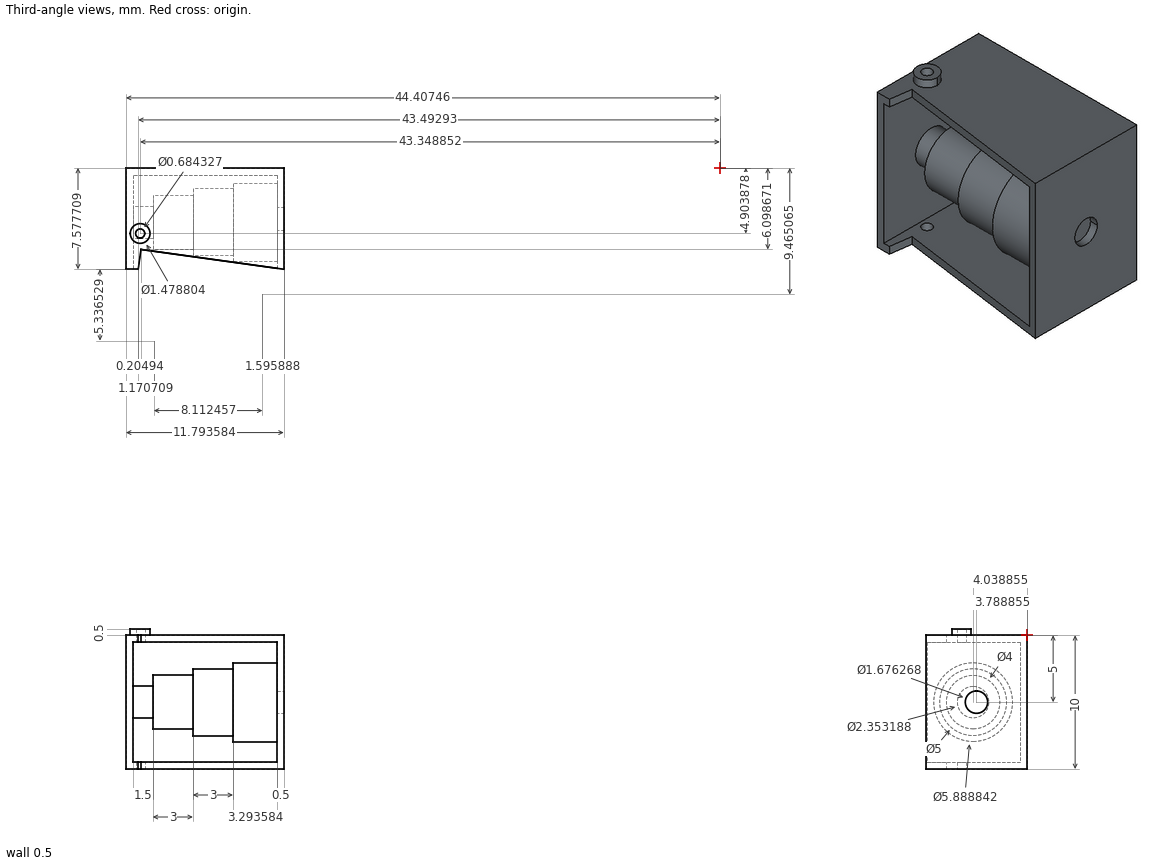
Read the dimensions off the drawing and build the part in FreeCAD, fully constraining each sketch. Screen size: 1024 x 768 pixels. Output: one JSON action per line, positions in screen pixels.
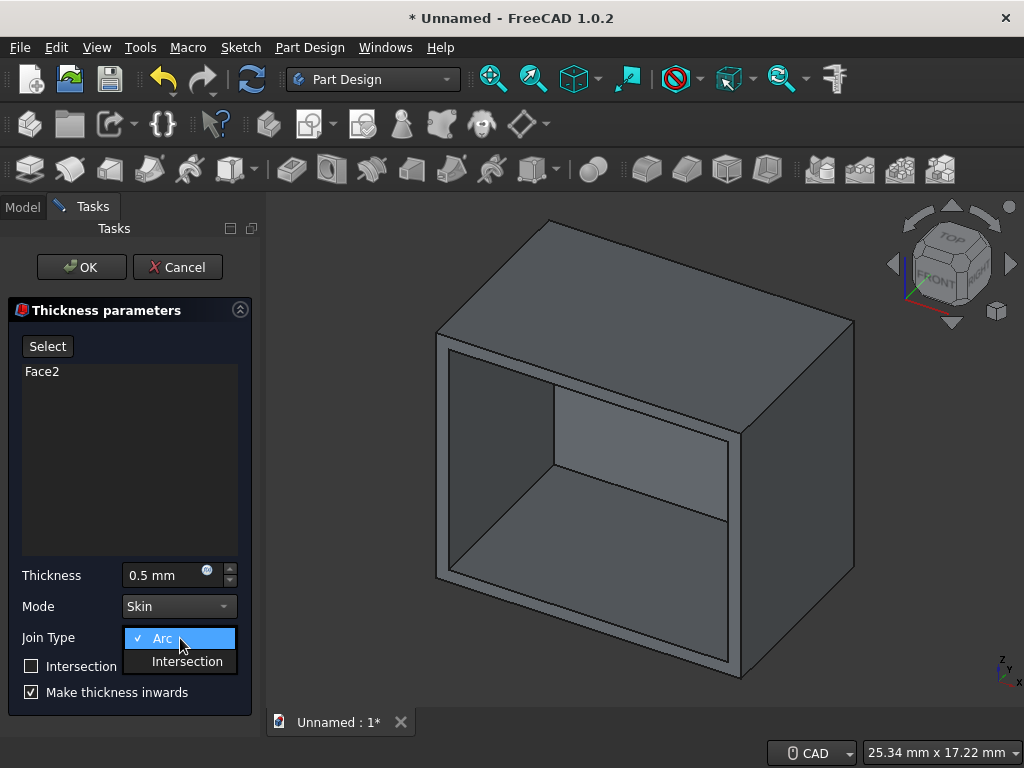
{"action": "left_click", "coordinate": [179, 662]}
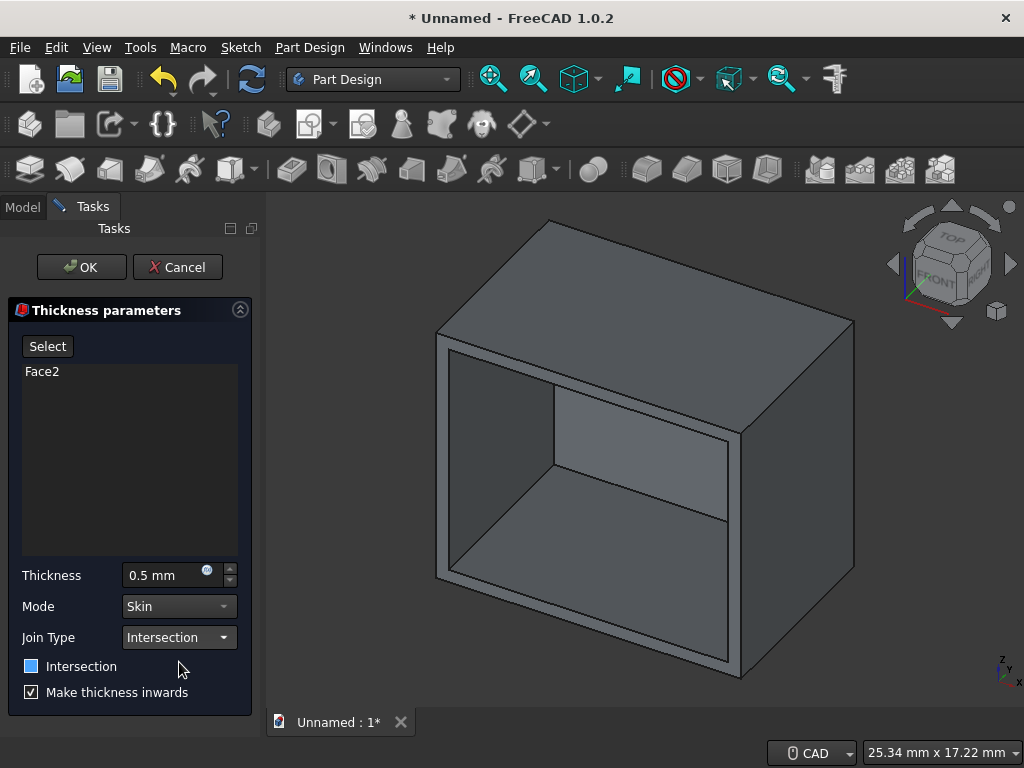
{"action": "left_click", "coordinate": [82, 267]}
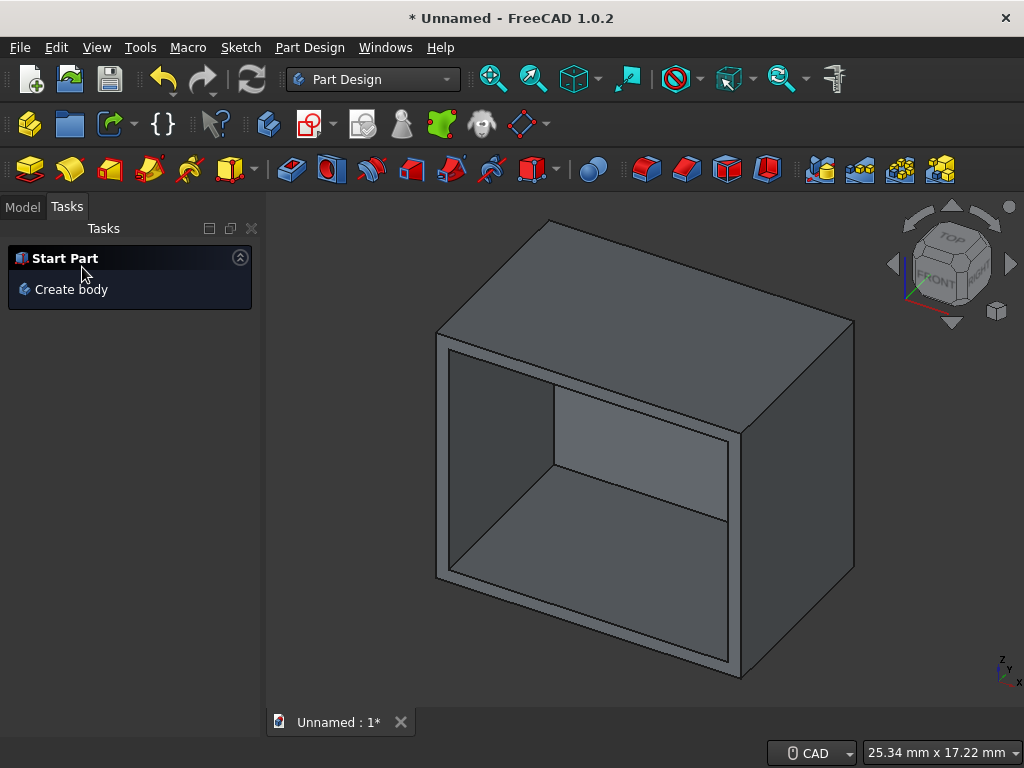
{"action": "left_click", "coordinate": [310, 124]}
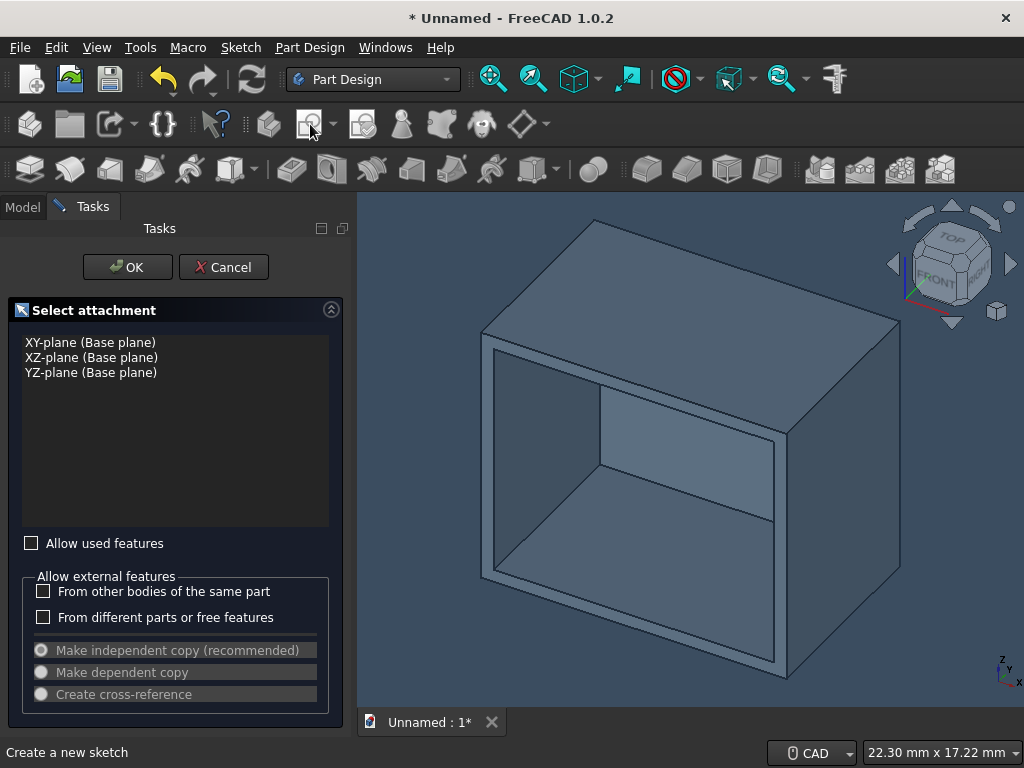
{"action": "left_click", "coordinate": [82, 342]}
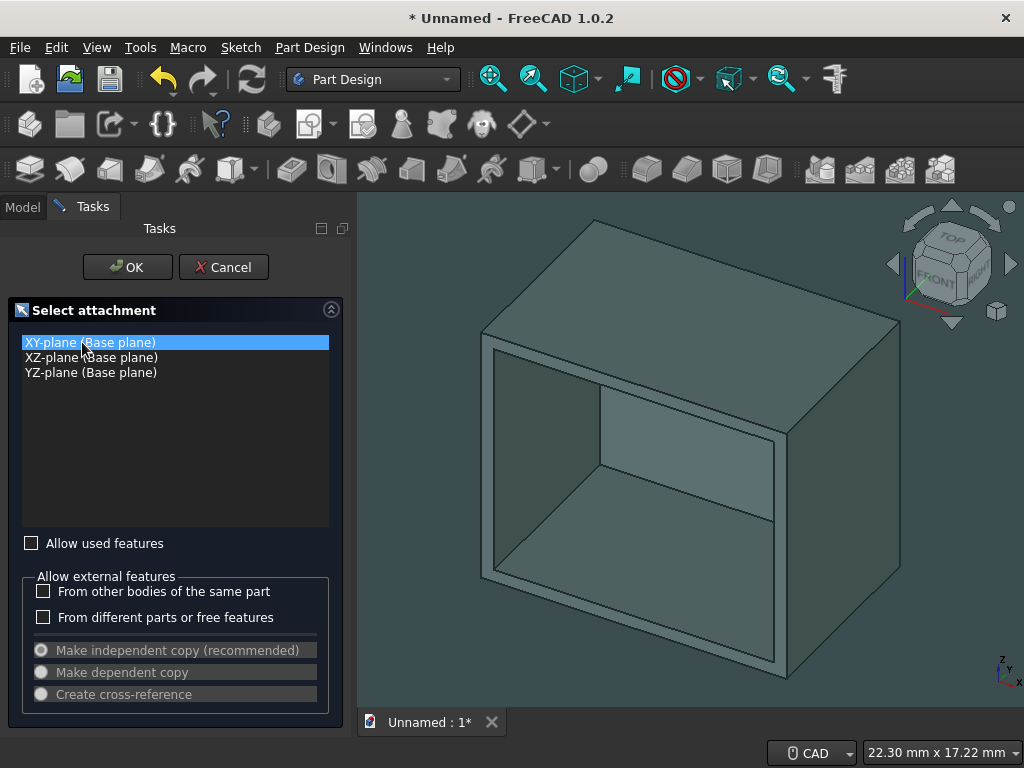
{"action": "left_click", "coordinate": [128, 267]}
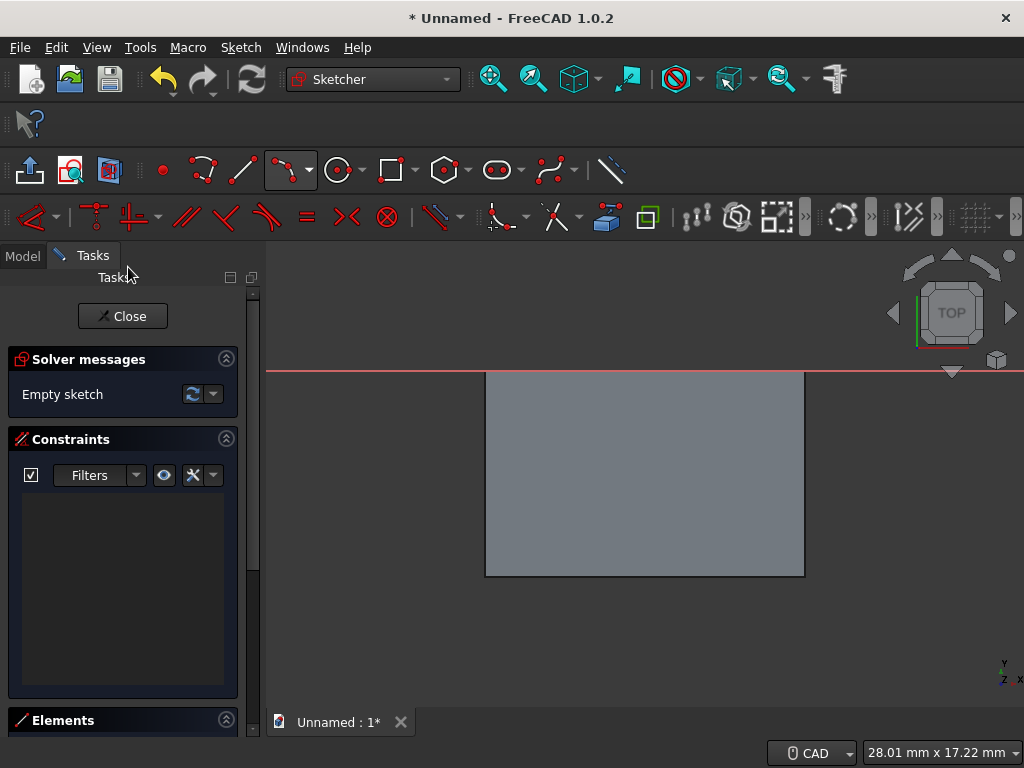
{"action": "scroll", "coordinate": [294, 269], "scroll_direction": "down", "scroll_amount": 1}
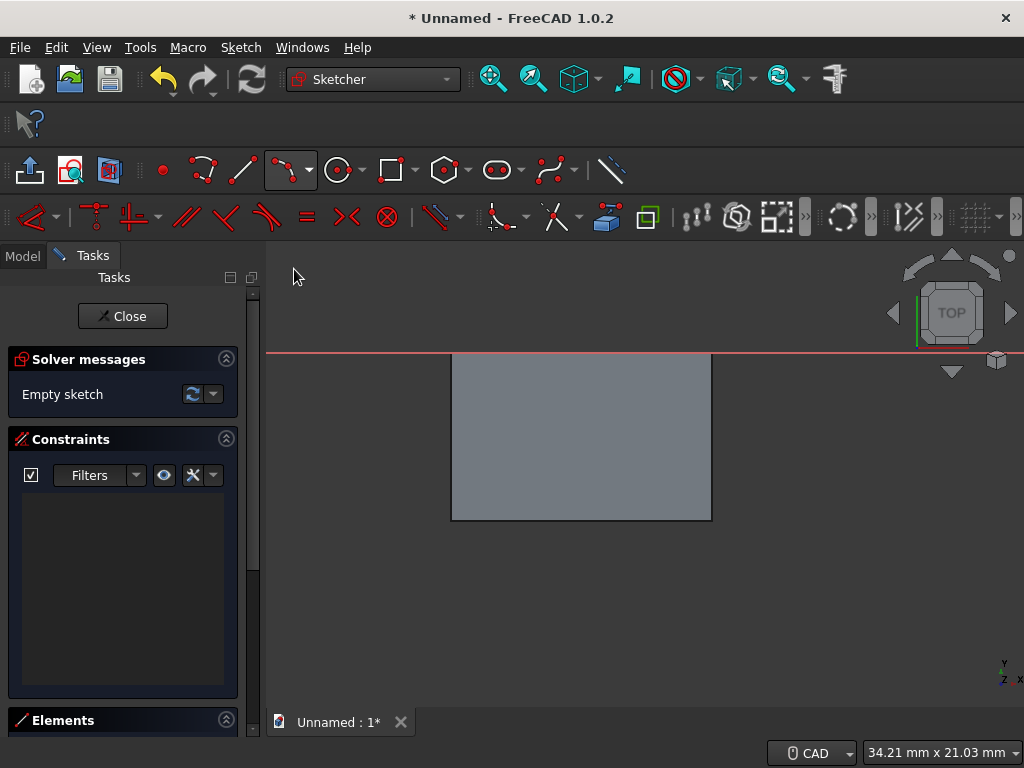
{"action": "scroll", "coordinate": [610, 672], "scroll_direction": "up", "scroll_amount": 3}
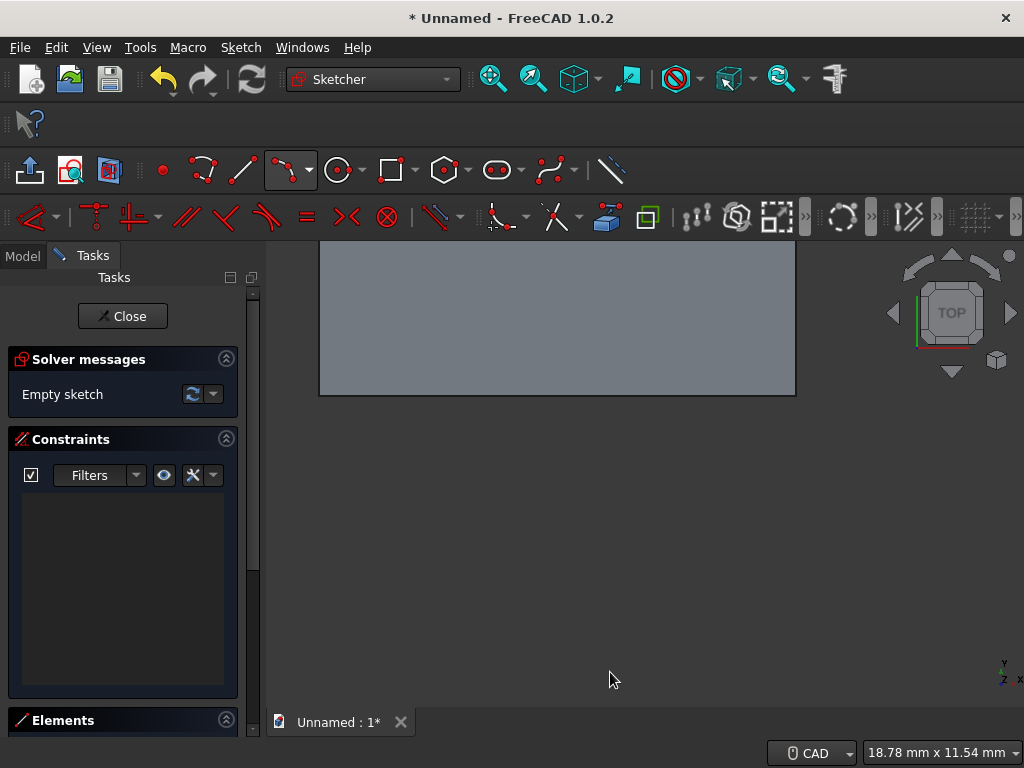
{"action": "left_click", "coordinate": [204, 170]}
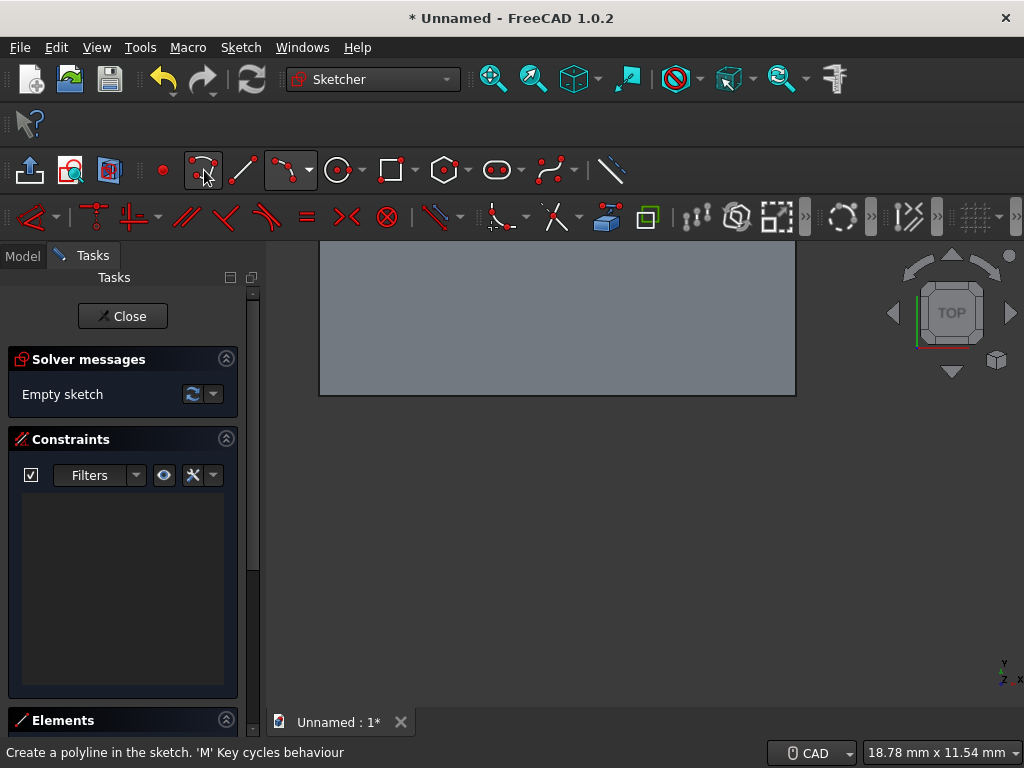
{"action": "left_click", "coordinate": [796, 396]}
{"action": "left_click", "coordinate": [365, 336]}
{"action": "left_click", "coordinate": [356, 396]}
{"action": "left_click", "coordinate": [404, 611]}
{"action": "left_click", "coordinate": [731, 472]}
{"action": "left_click", "coordinate": [796, 397]}
{"action": "key", "text": "Escape"}
{"action": "key", "text": "Escape"}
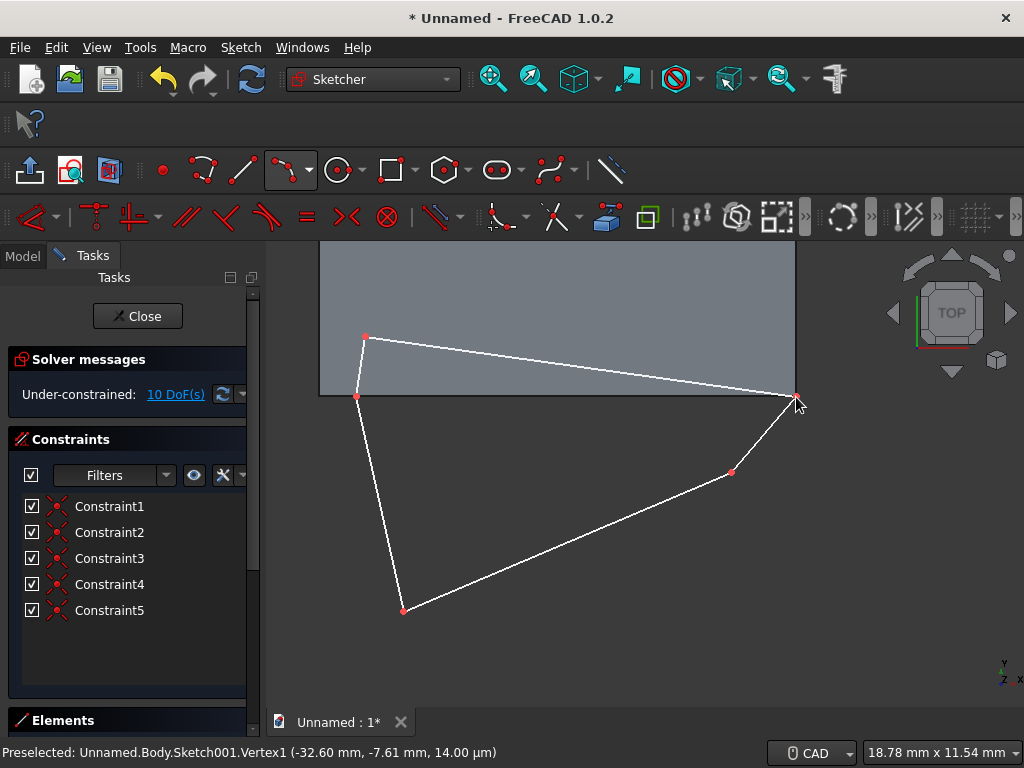
{"action": "left_click", "coordinate": [32, 218]}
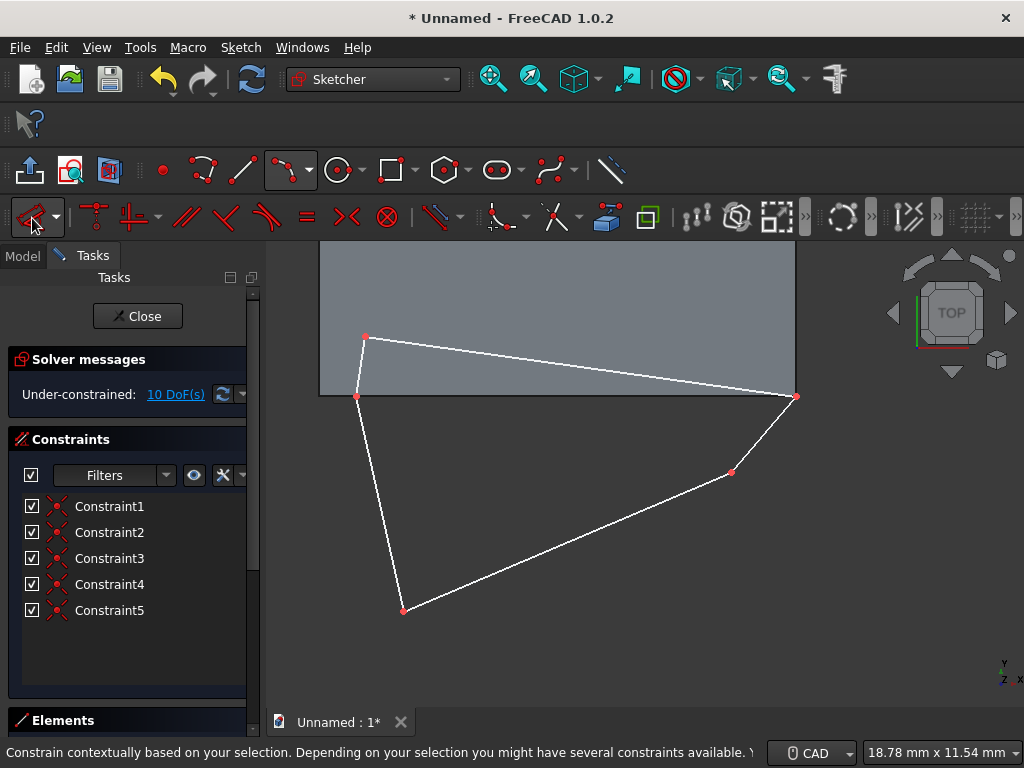
{"action": "scroll", "coordinate": [362, 355], "scroll_direction": "up", "scroll_amount": 8}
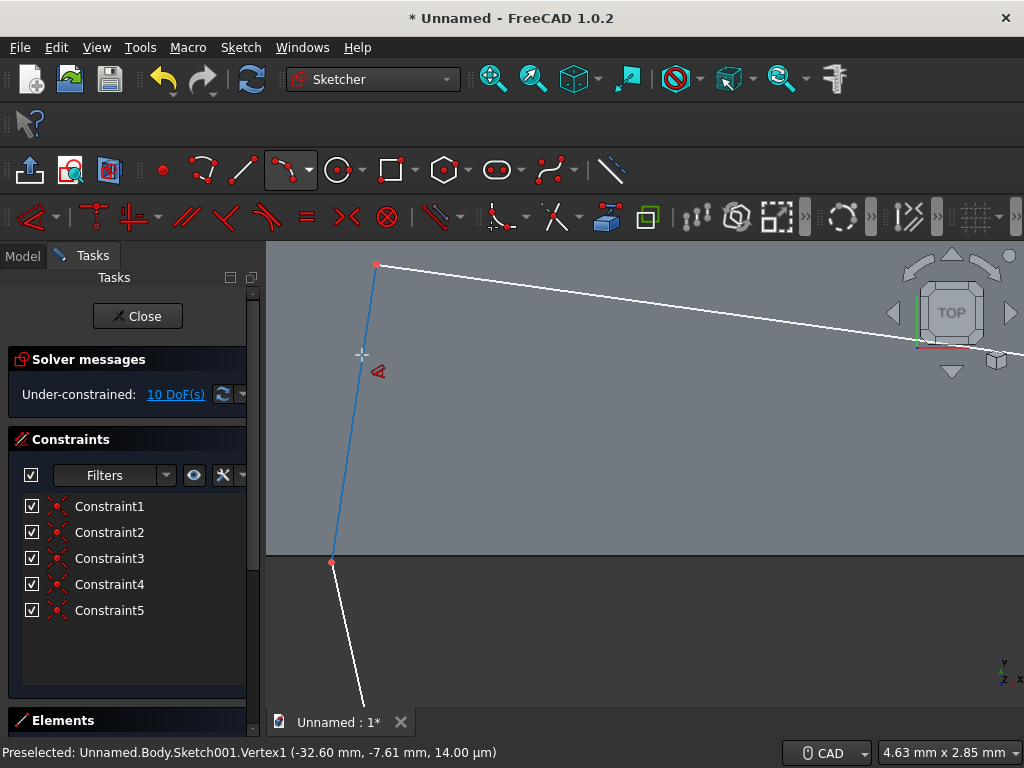
{"action": "left_click", "coordinate": [363, 354]}
{"action": "left_click", "coordinate": [354, 596]}